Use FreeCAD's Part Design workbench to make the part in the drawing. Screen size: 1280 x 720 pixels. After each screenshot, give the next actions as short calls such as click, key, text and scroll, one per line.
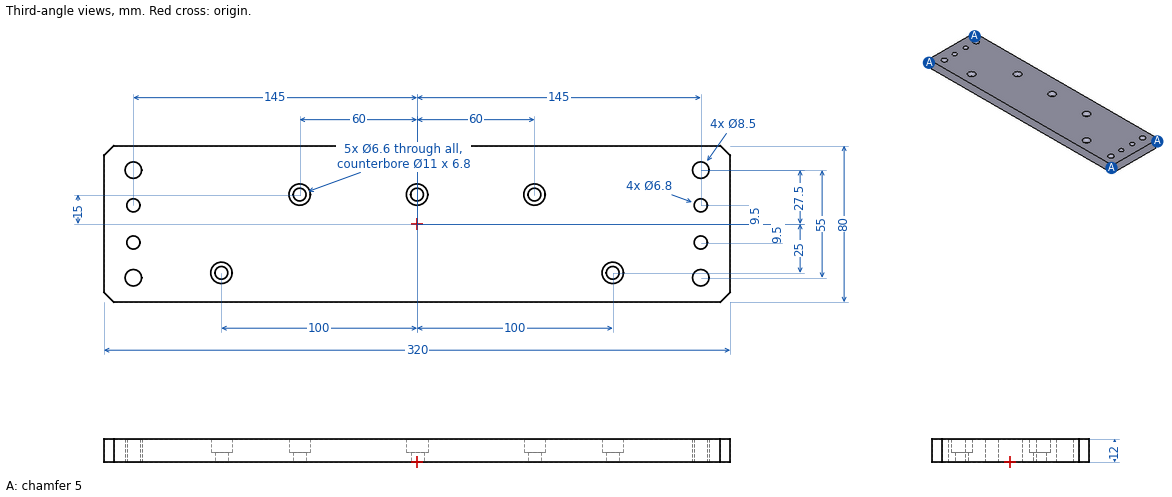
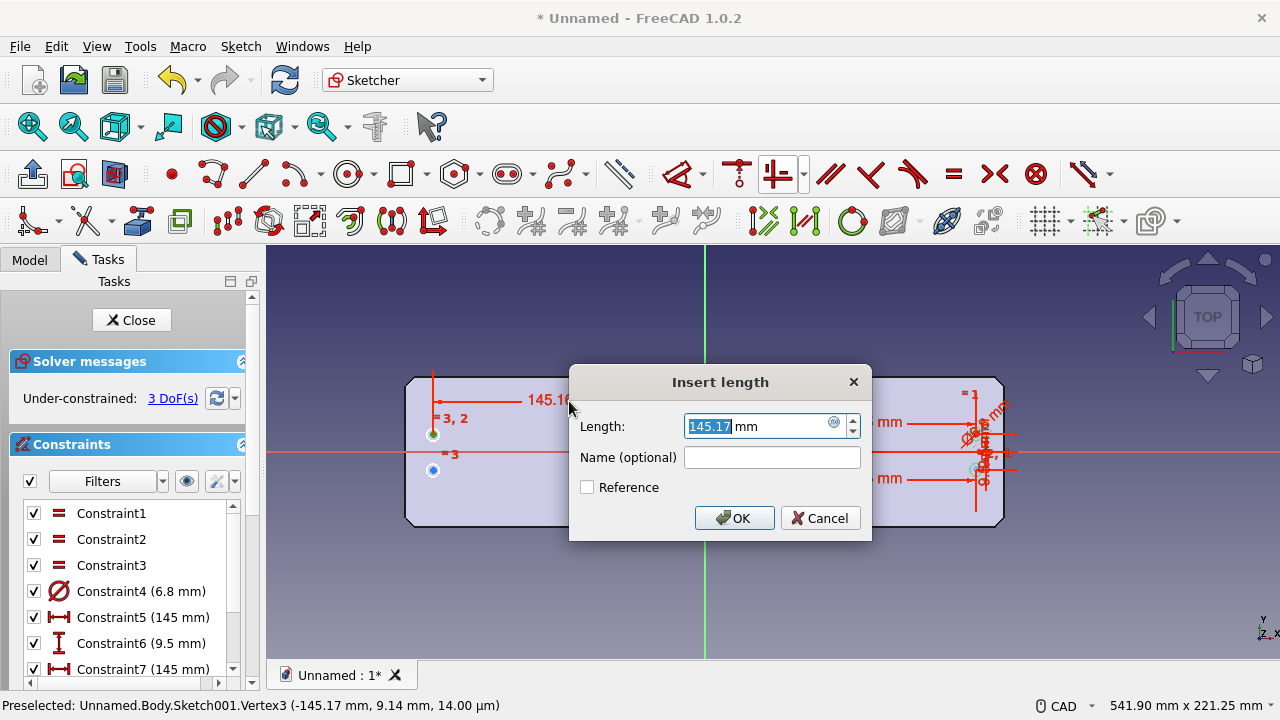
text(145)
key(Return)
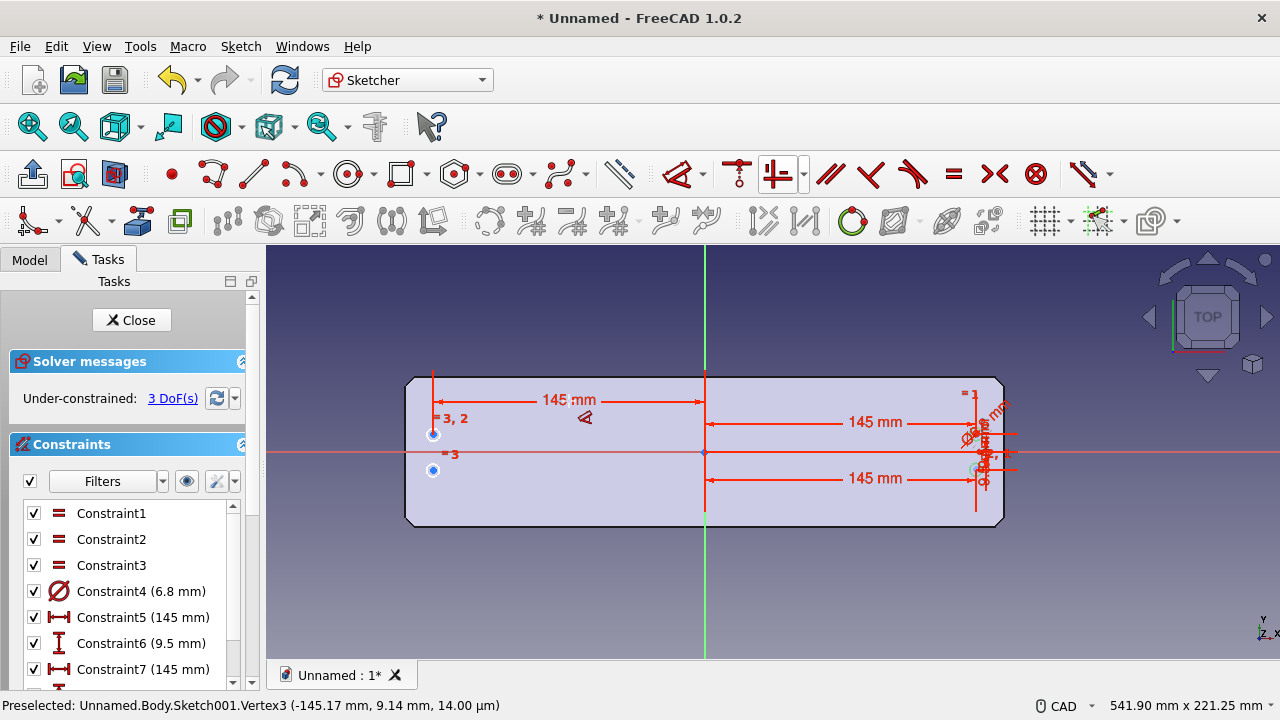
scroll(433, 435, up, 5)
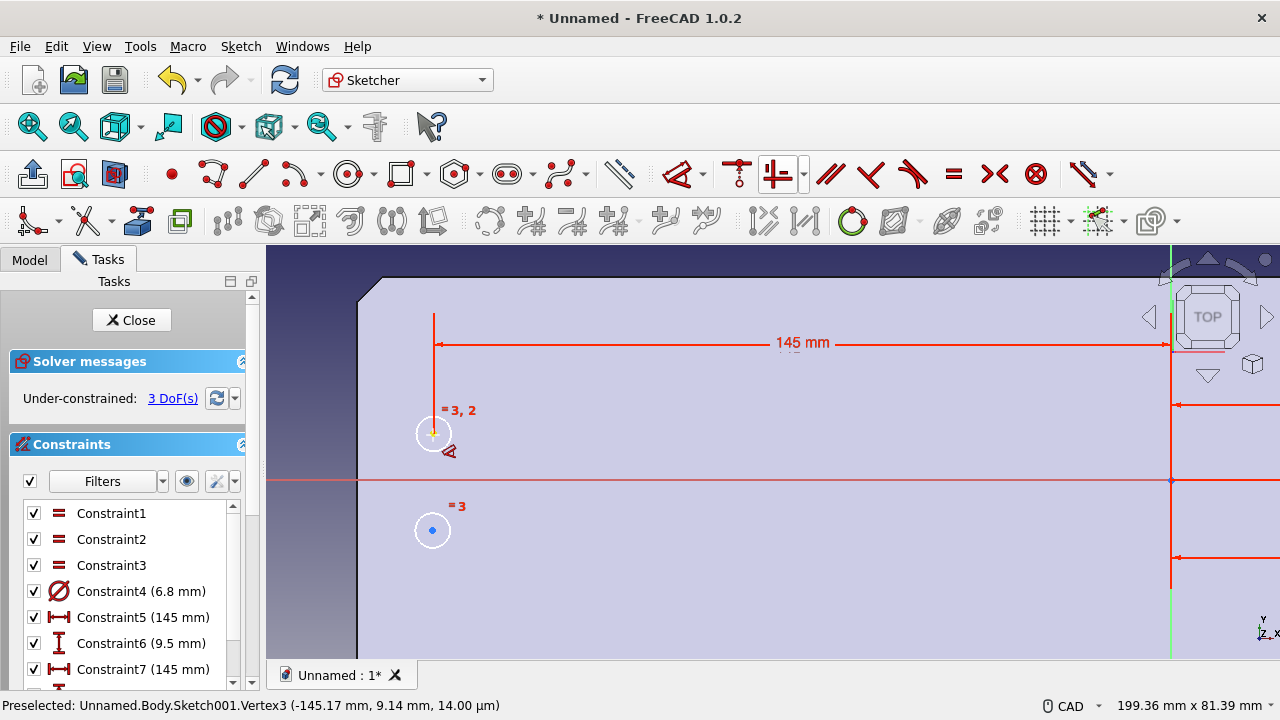
click(434, 434)
click(400, 457)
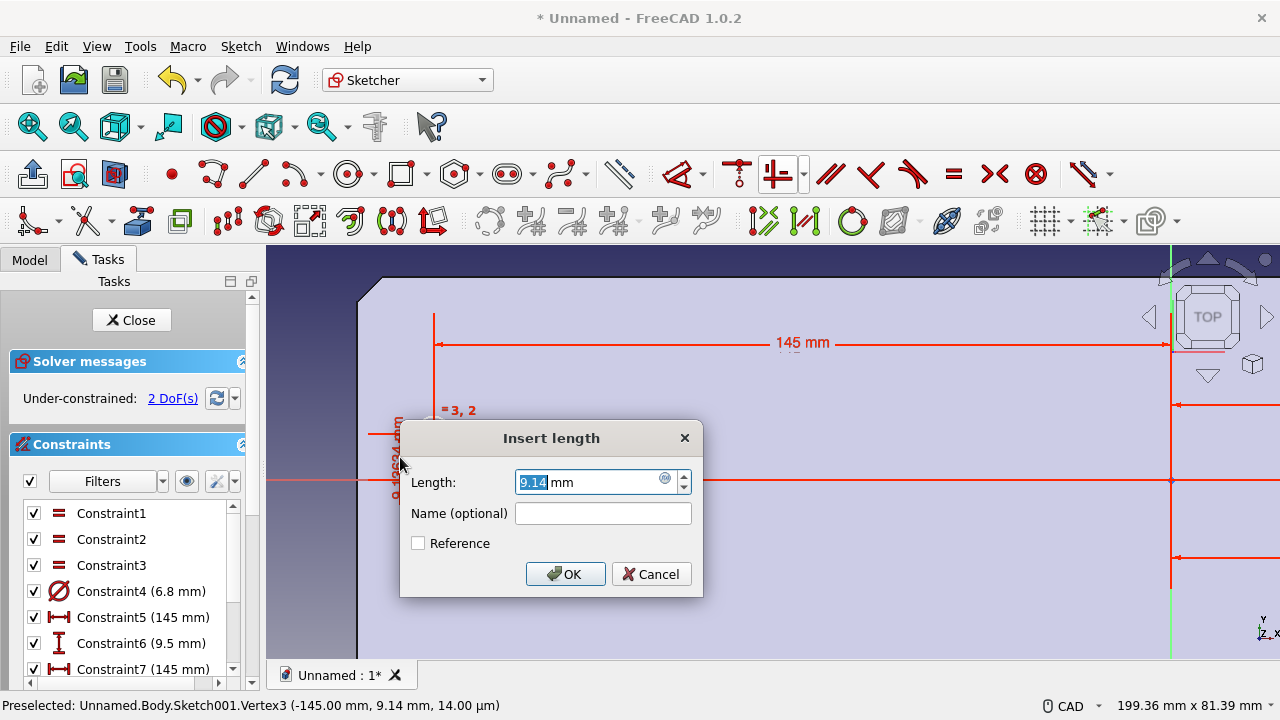
text(9.5)
key(Return)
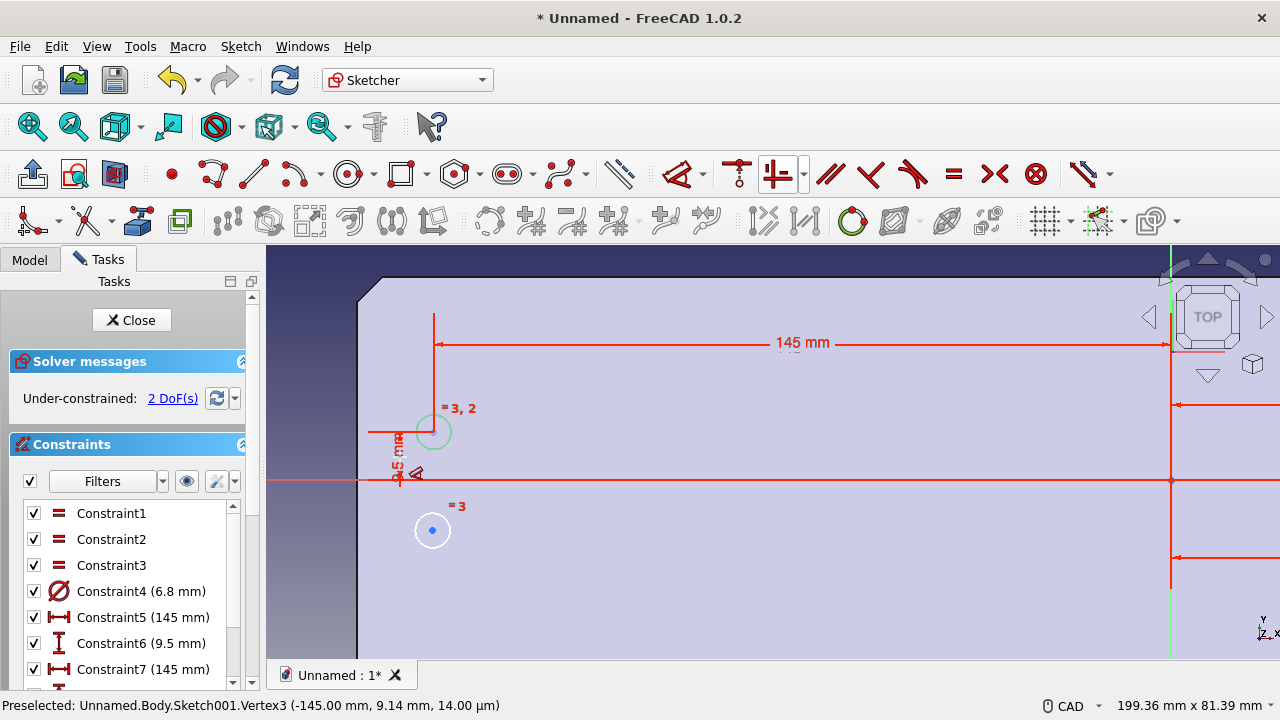
click(433, 531)
click(774, 565)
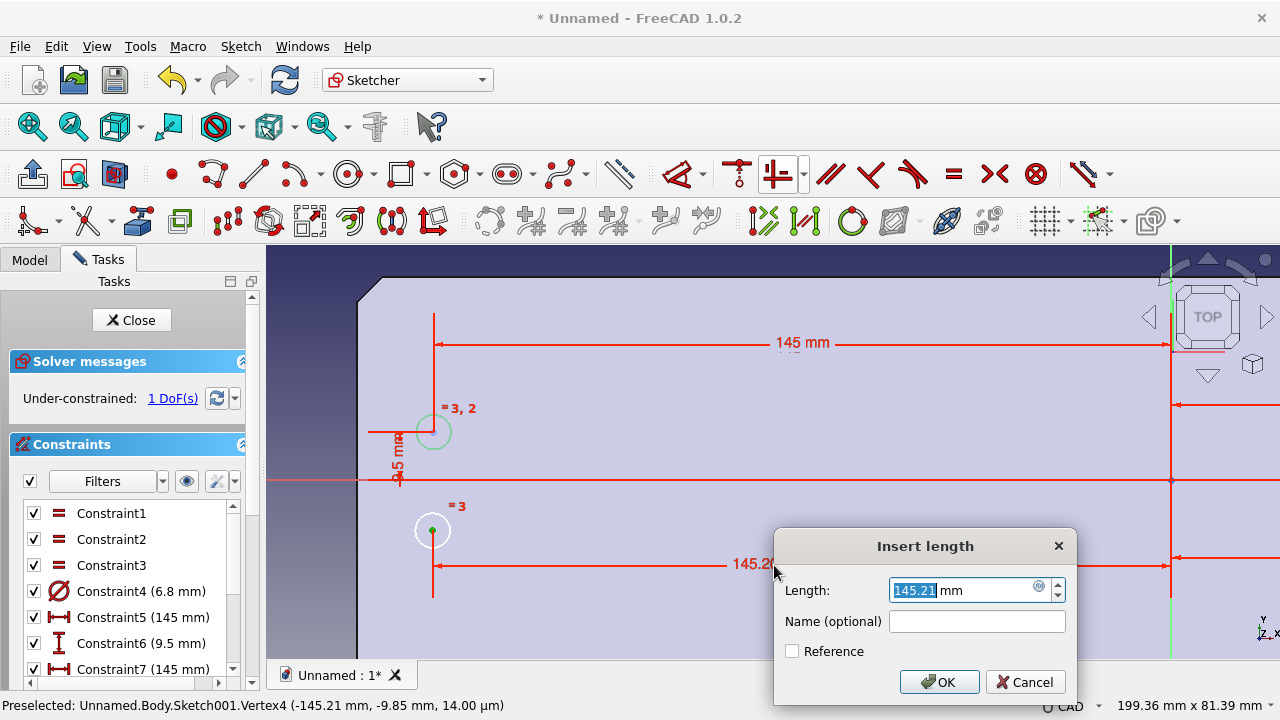
text(145)
key(Return)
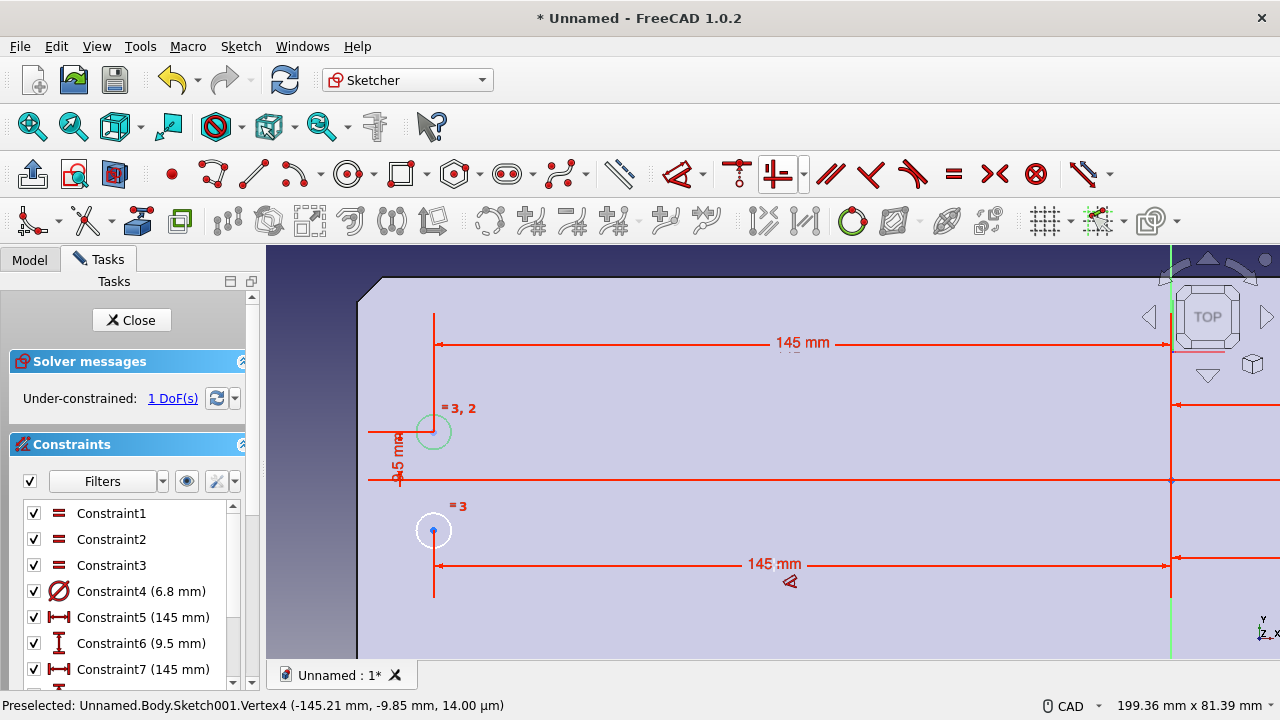
click(434, 531)
click(400, 506)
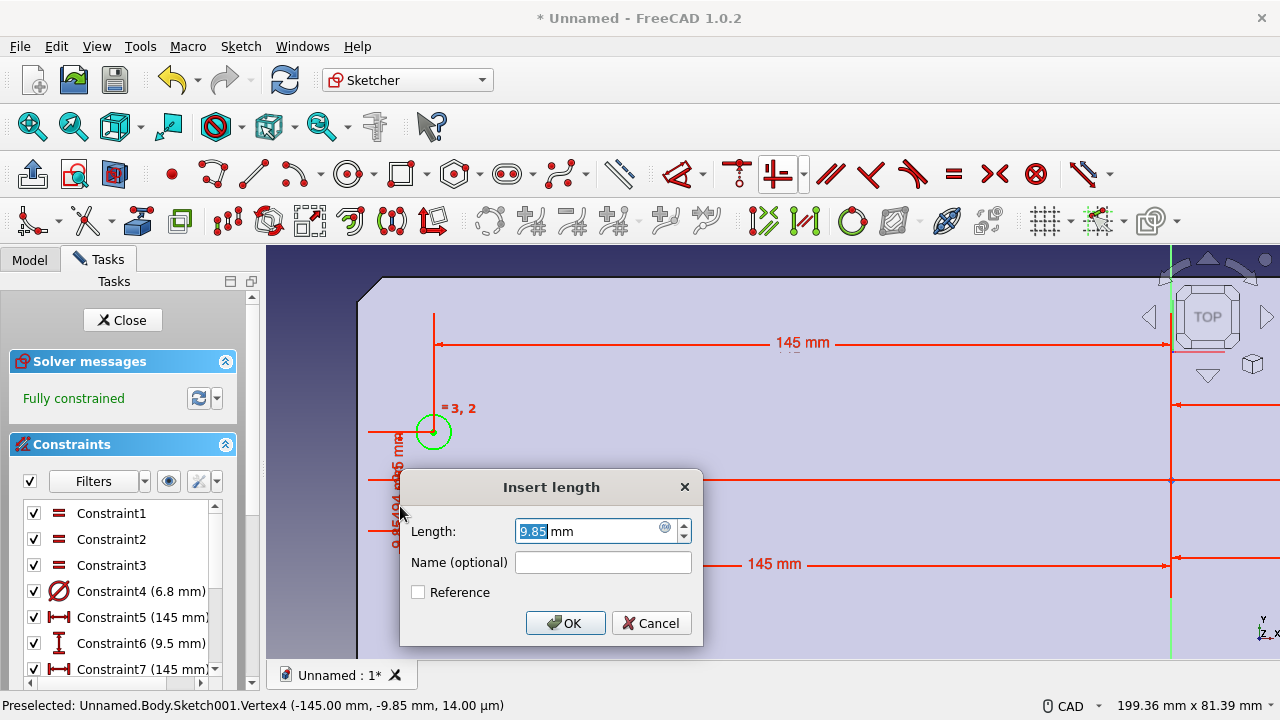
text(9.5)
key(Return)
key(Escape)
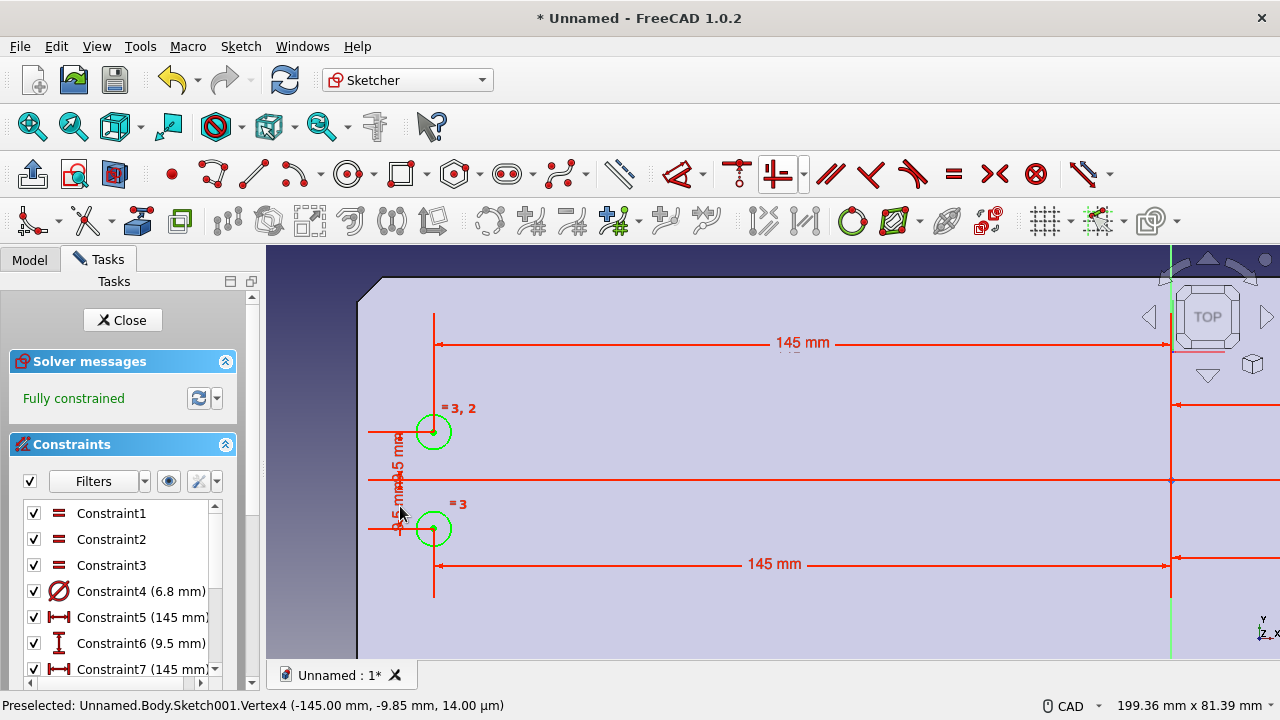
click(123, 320)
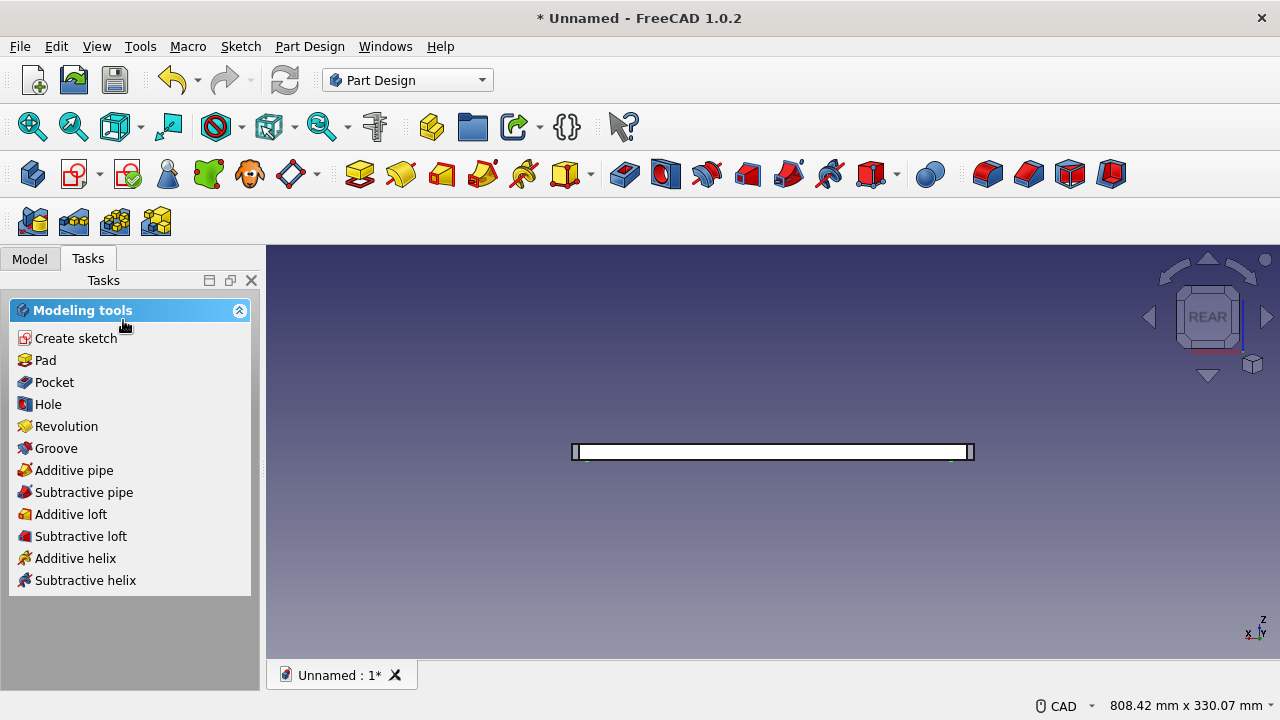
click(625, 174)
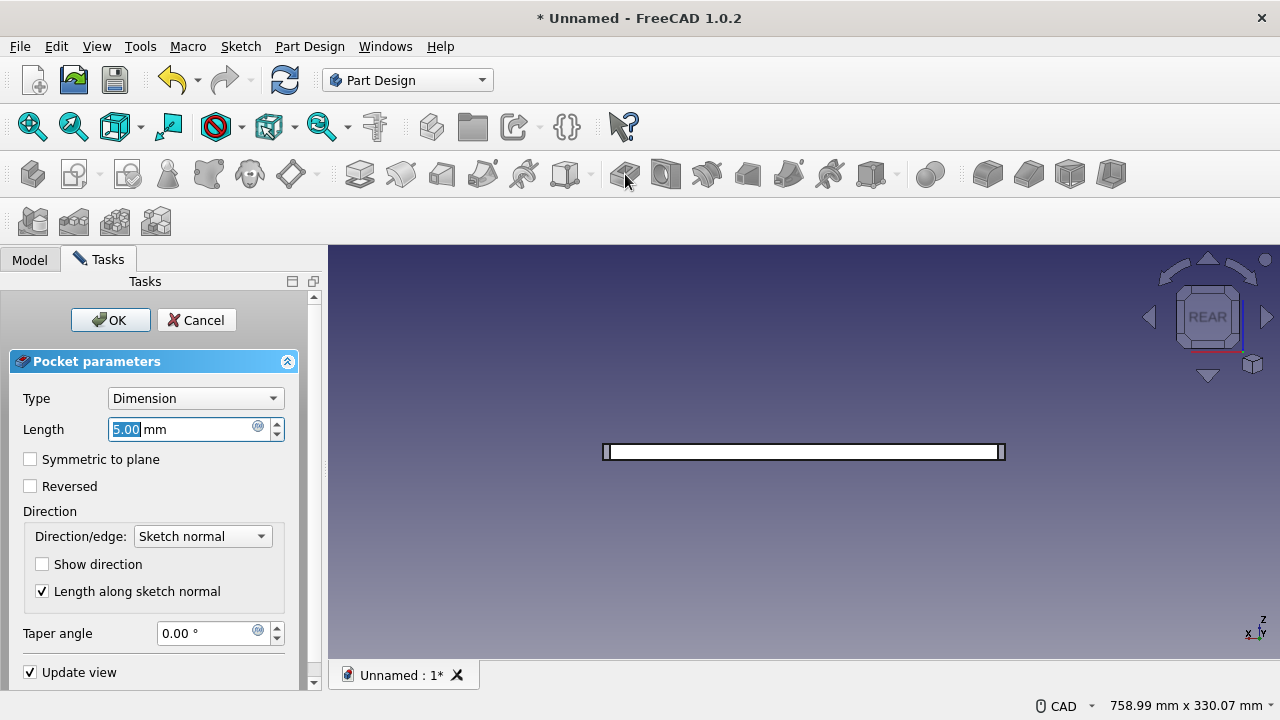
click(196, 398)